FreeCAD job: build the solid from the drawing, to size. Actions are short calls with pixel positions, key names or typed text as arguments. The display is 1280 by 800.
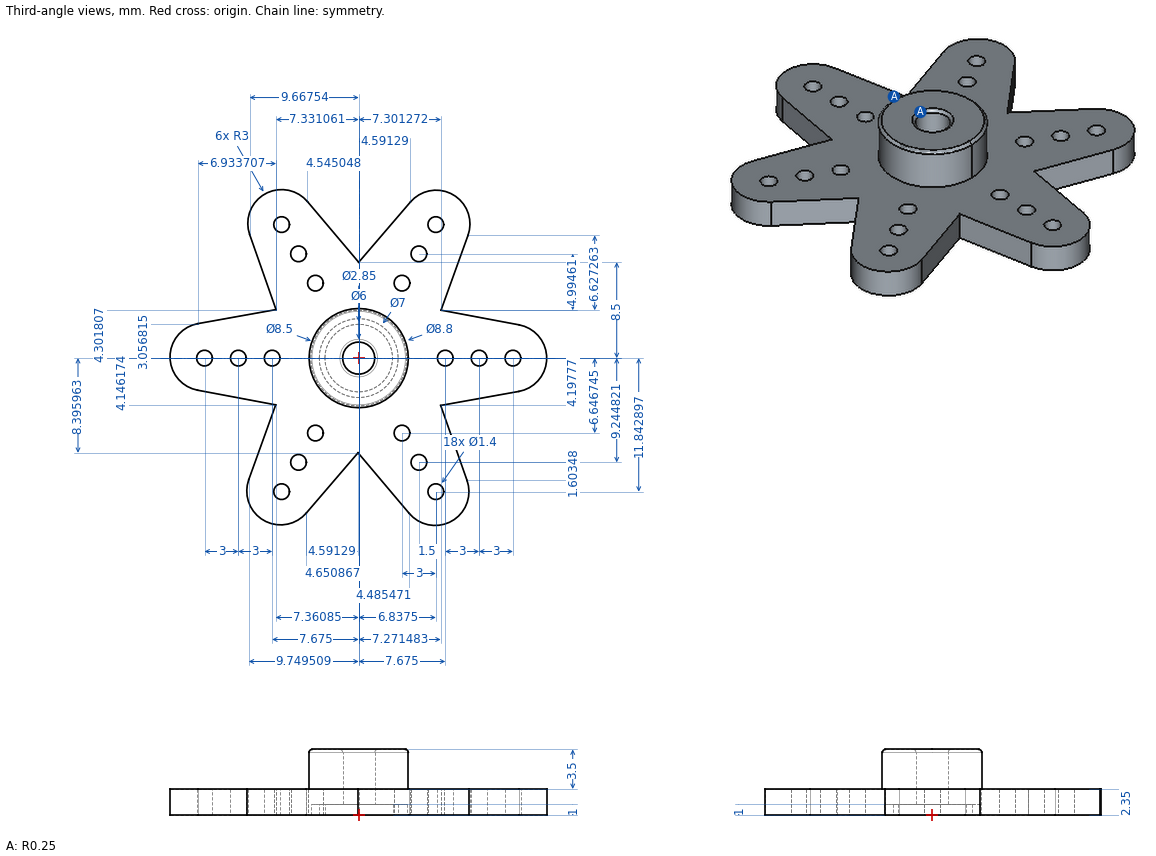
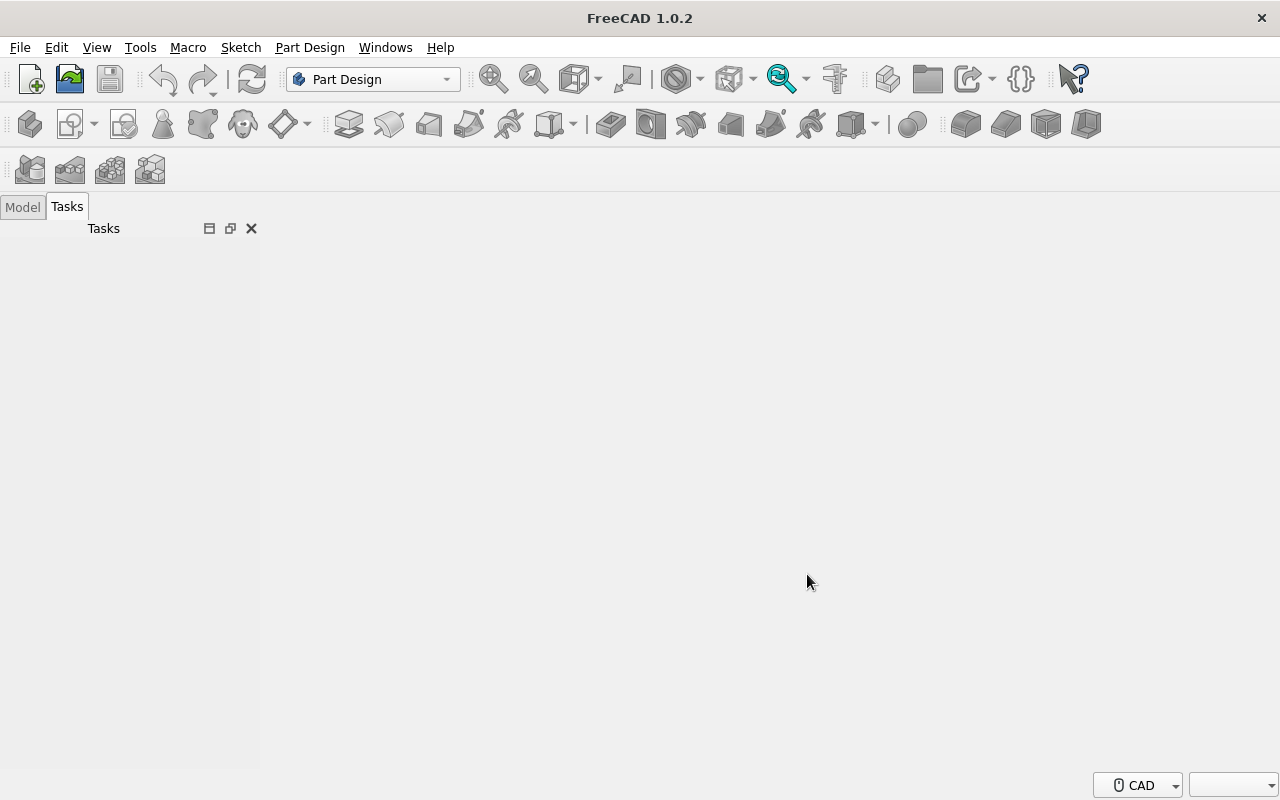
click(30, 80)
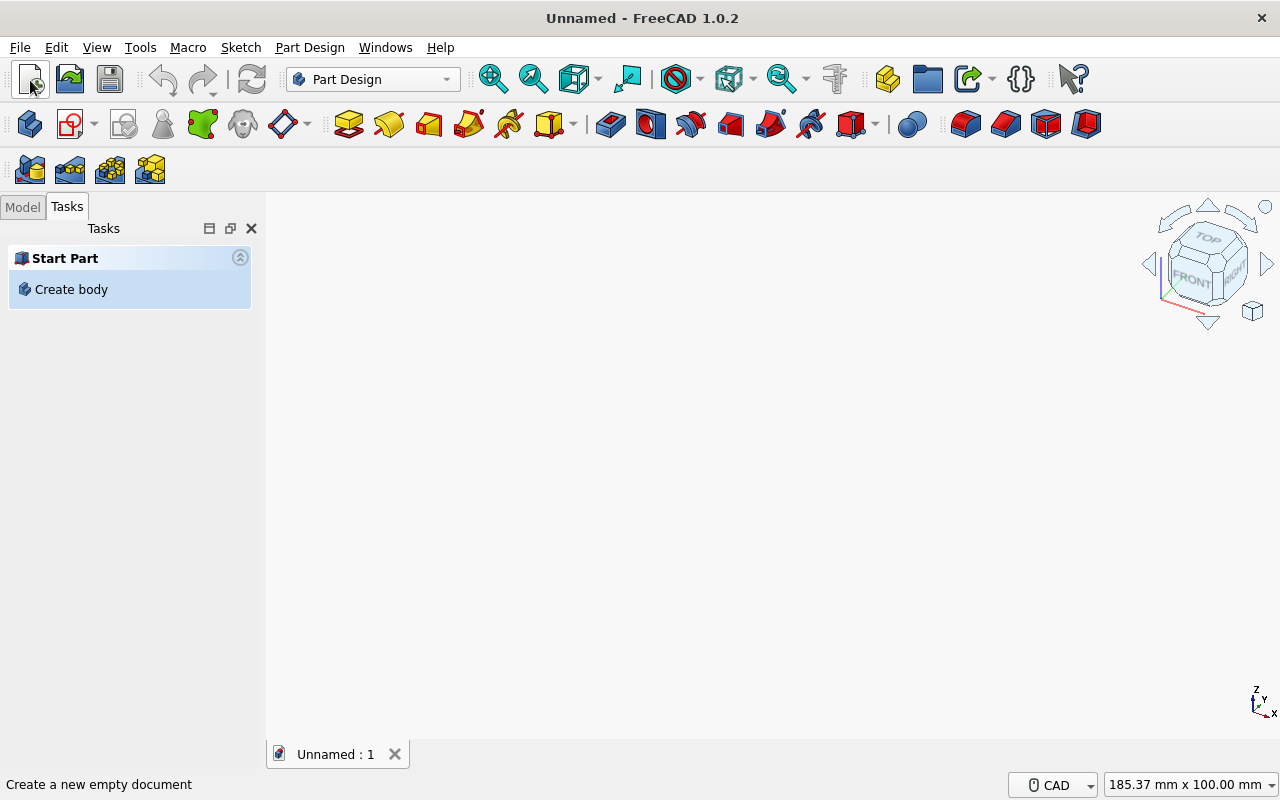
click(70, 124)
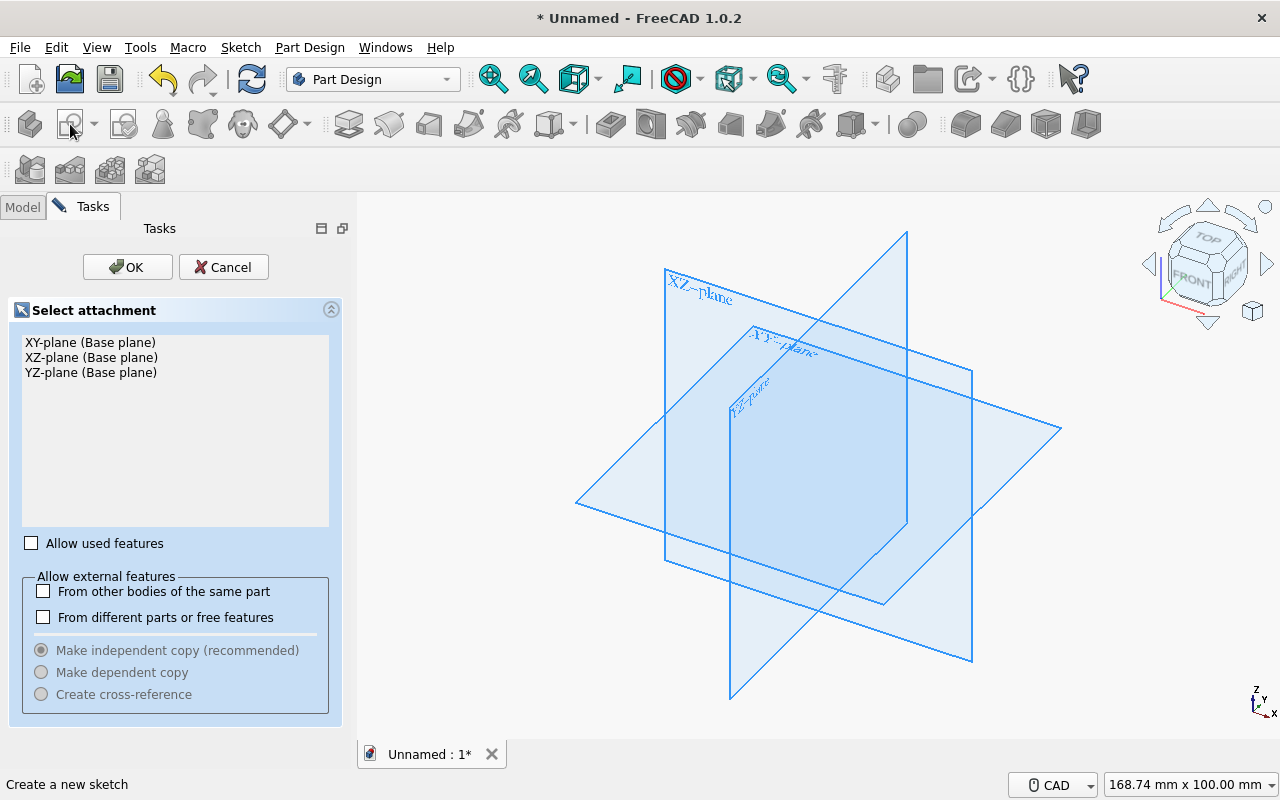
click(82, 342)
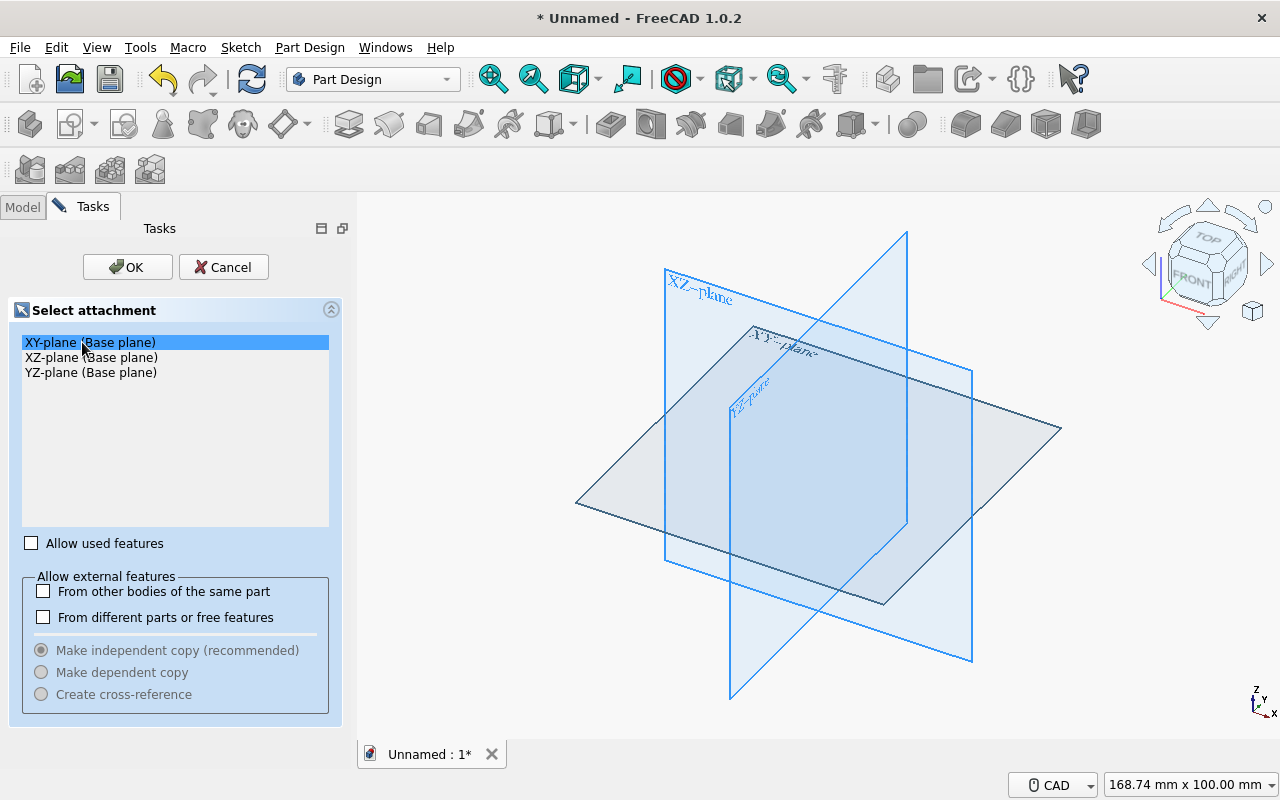
click(128, 267)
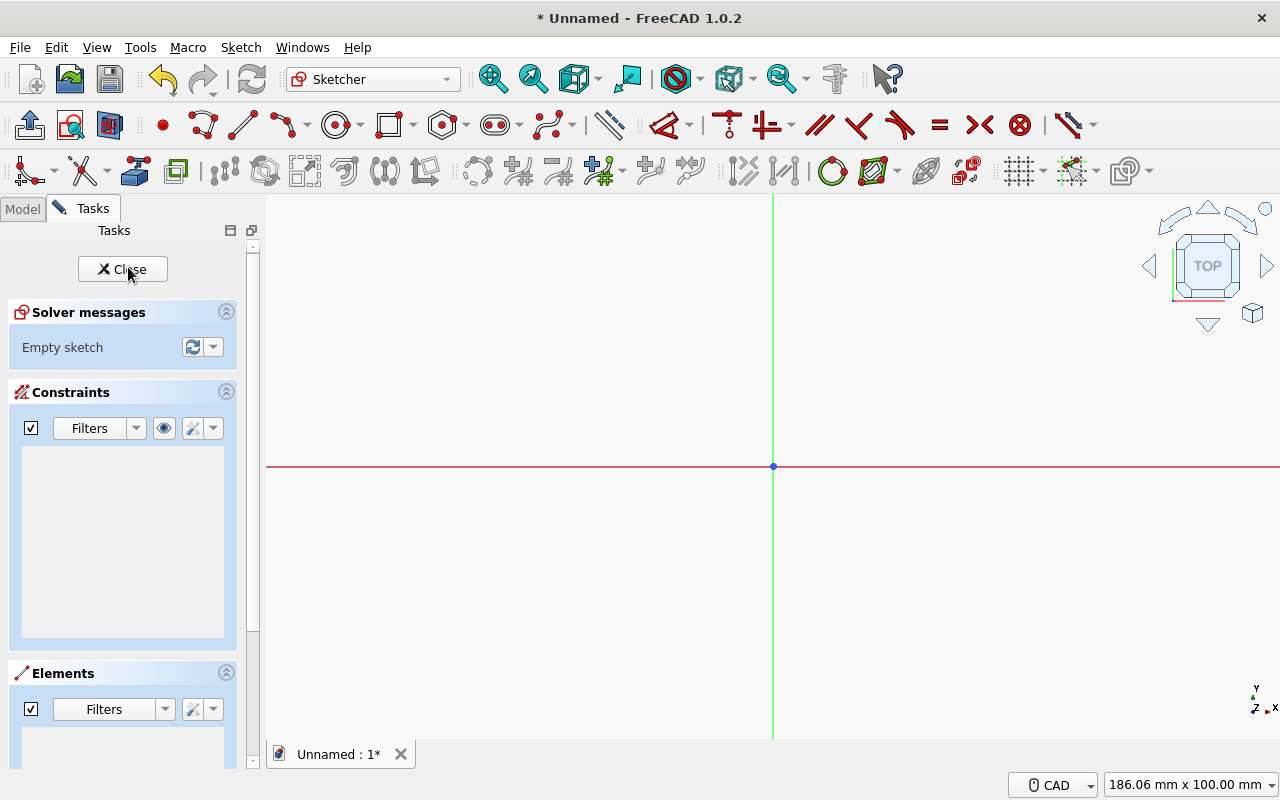
scroll(829, 466, up, 4)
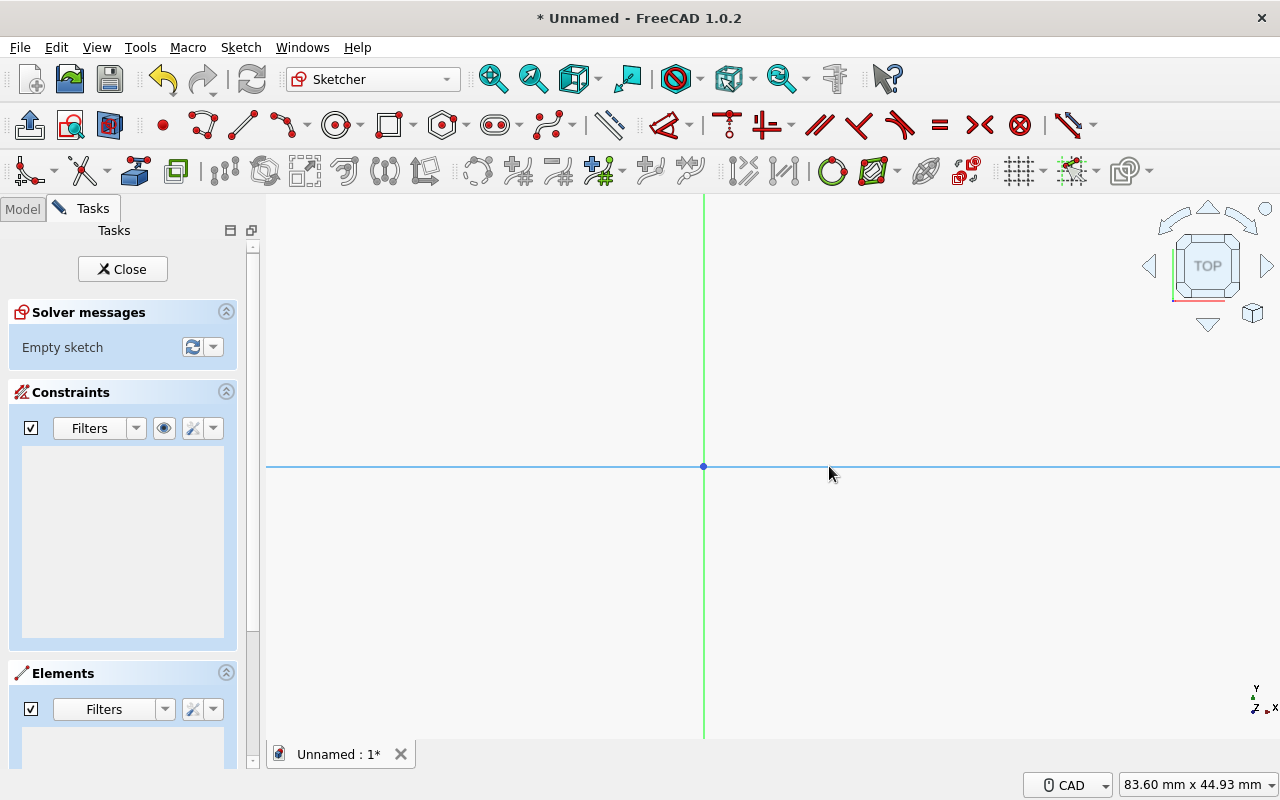
click(204, 126)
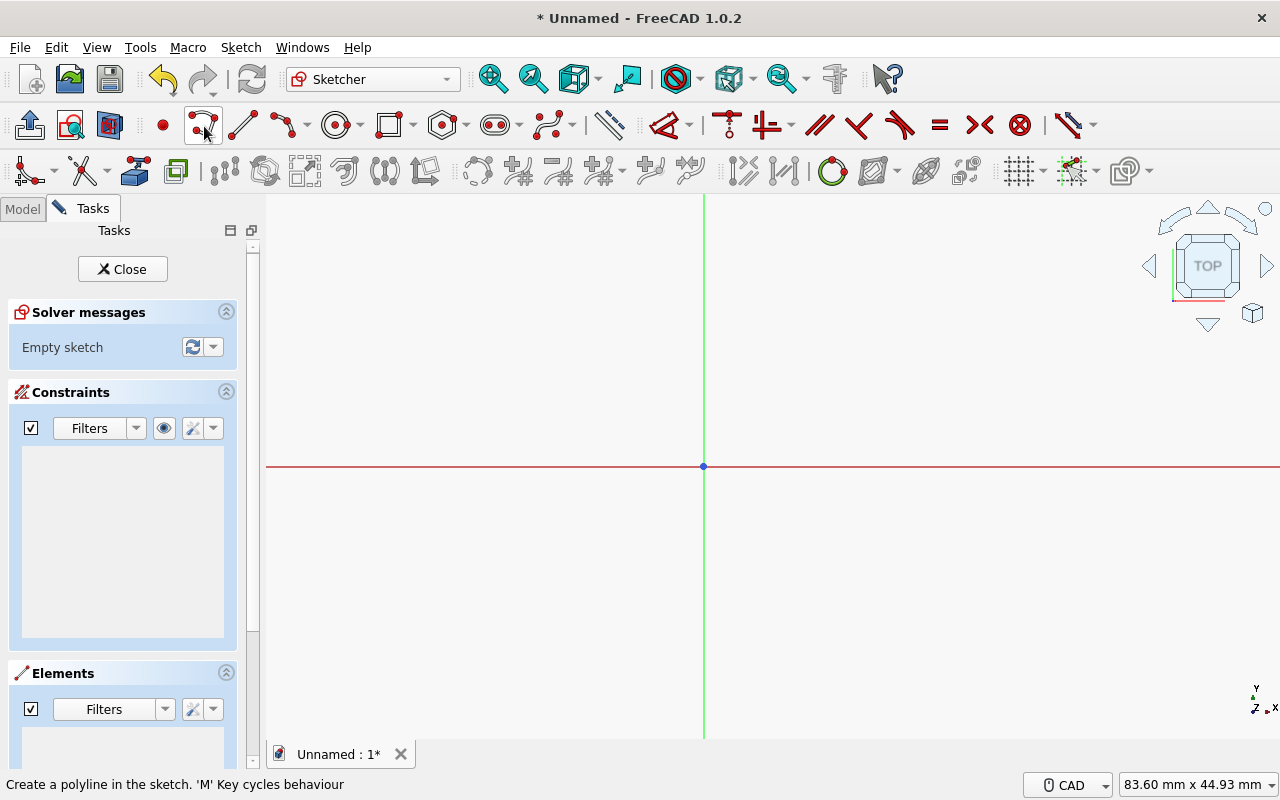
click(586, 334)
click(615, 414)
click(531, 429)
right_click(531, 429)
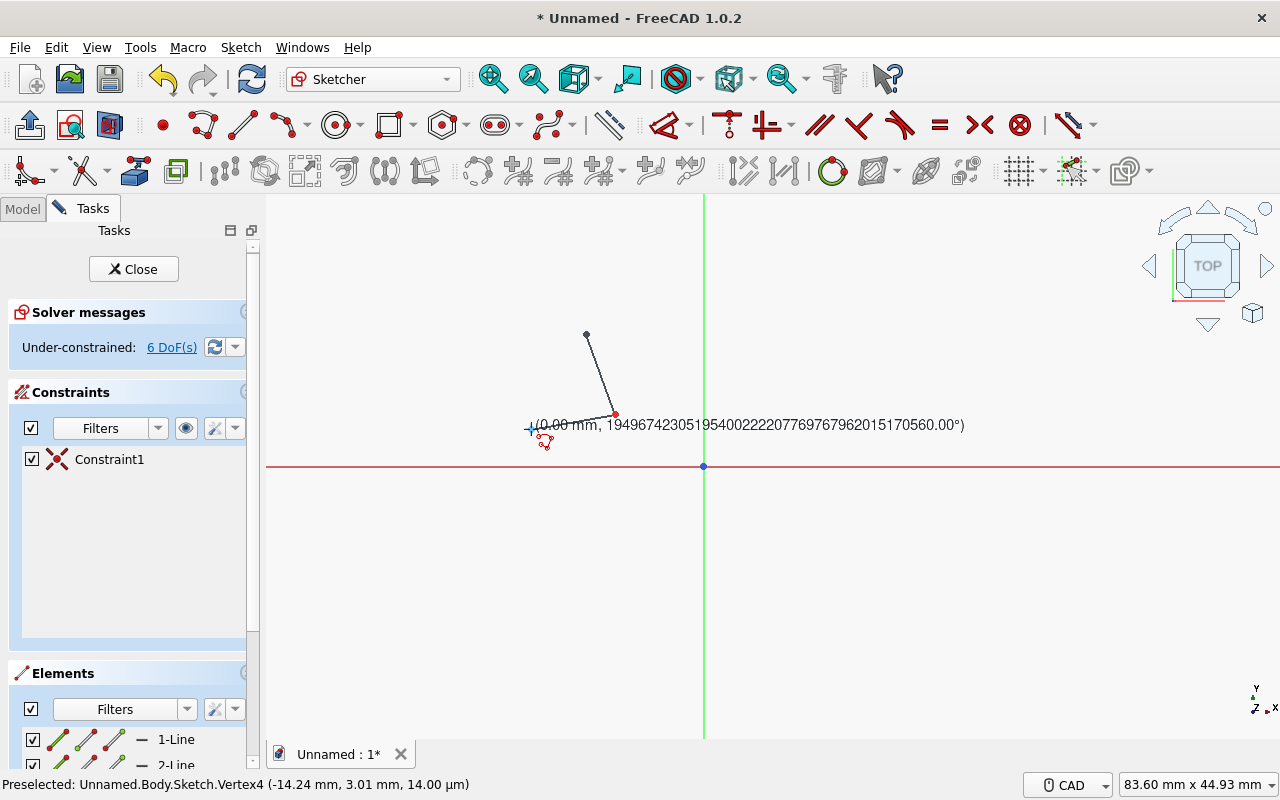
click(530, 501)
click(614, 517)
click(585, 597)
right_click(585, 597)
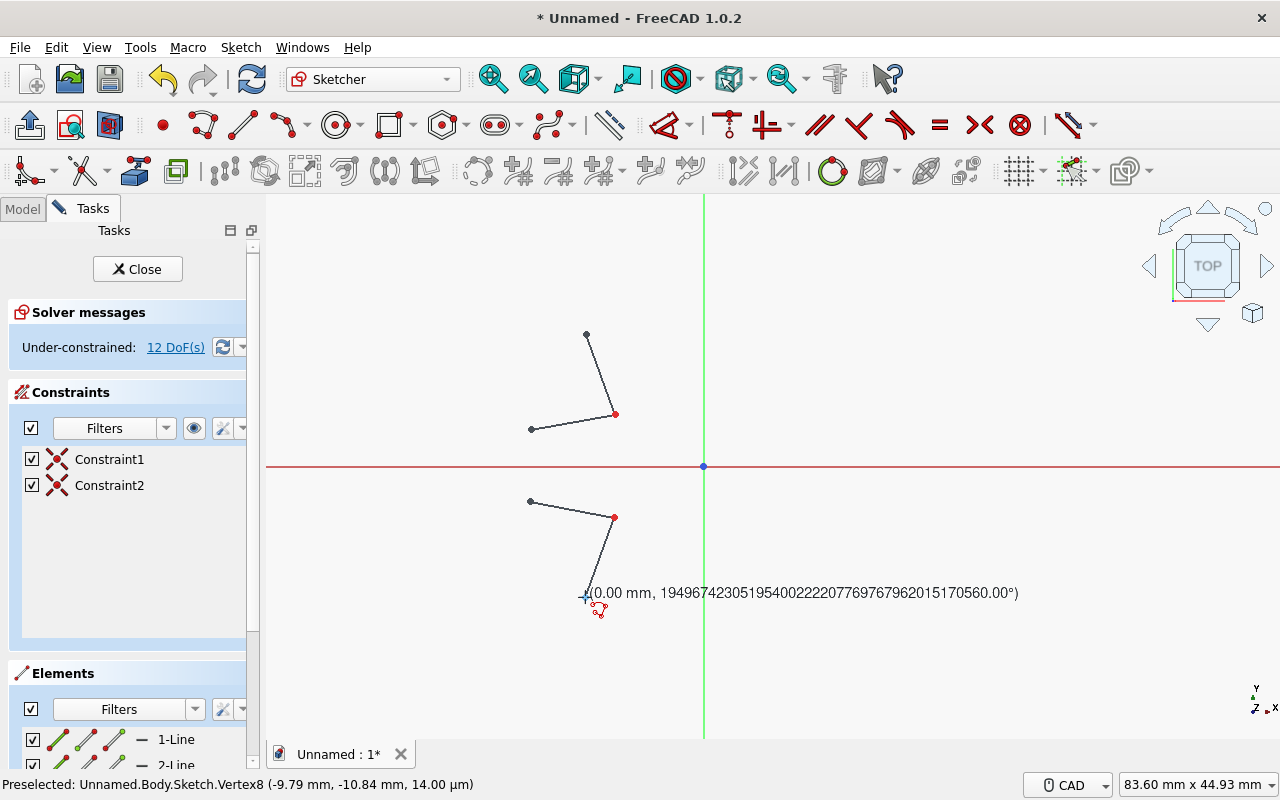
click(647, 633)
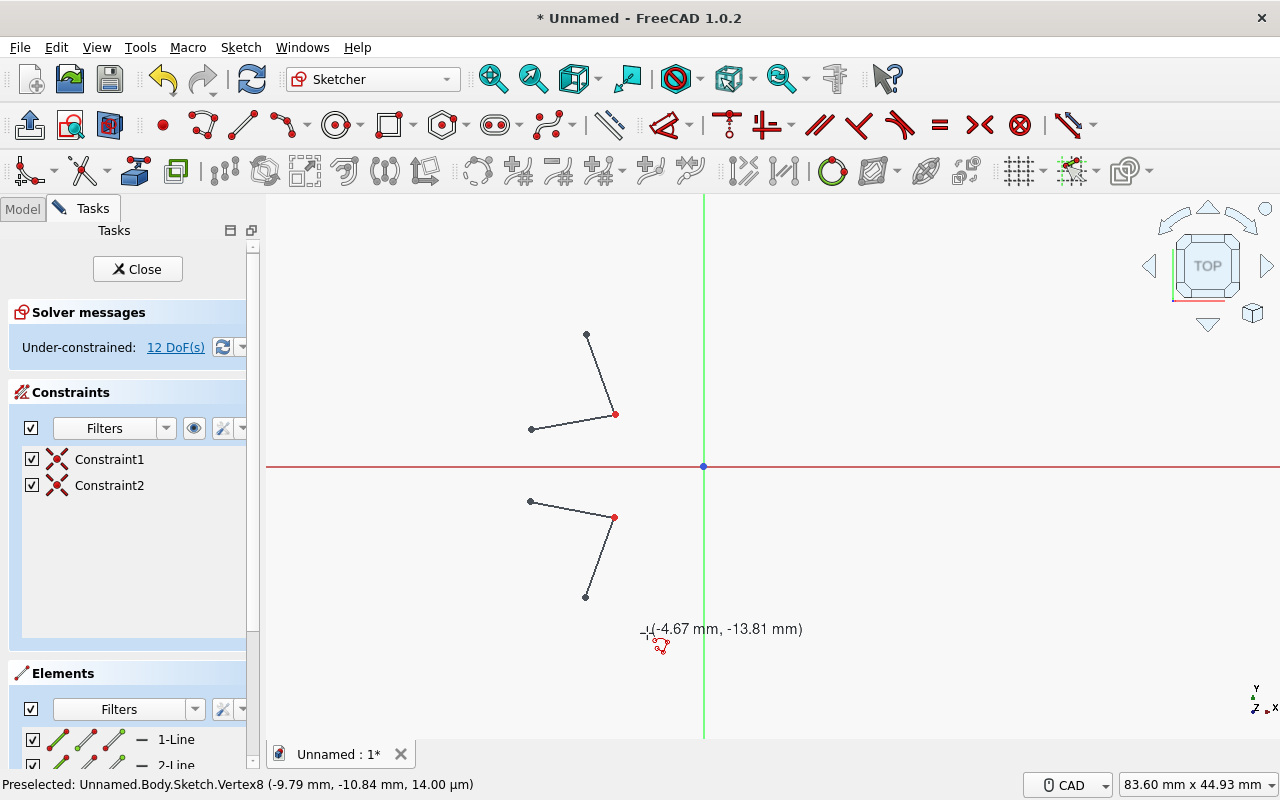
scroll(703, 568, up, 16)